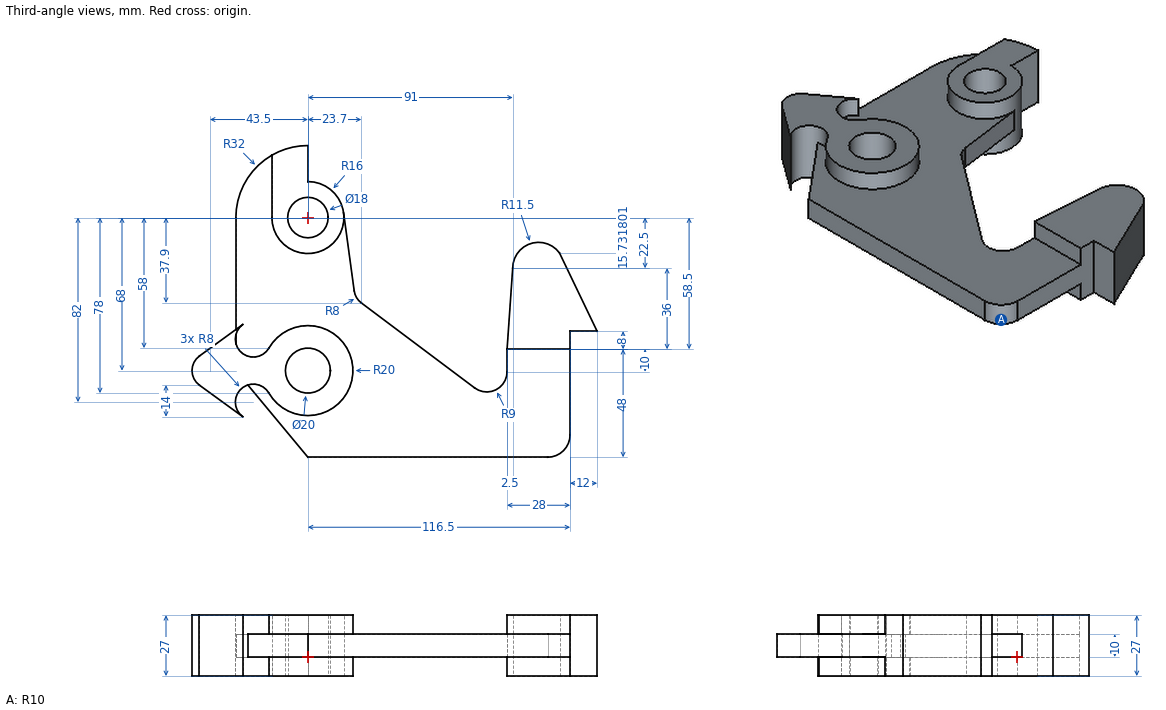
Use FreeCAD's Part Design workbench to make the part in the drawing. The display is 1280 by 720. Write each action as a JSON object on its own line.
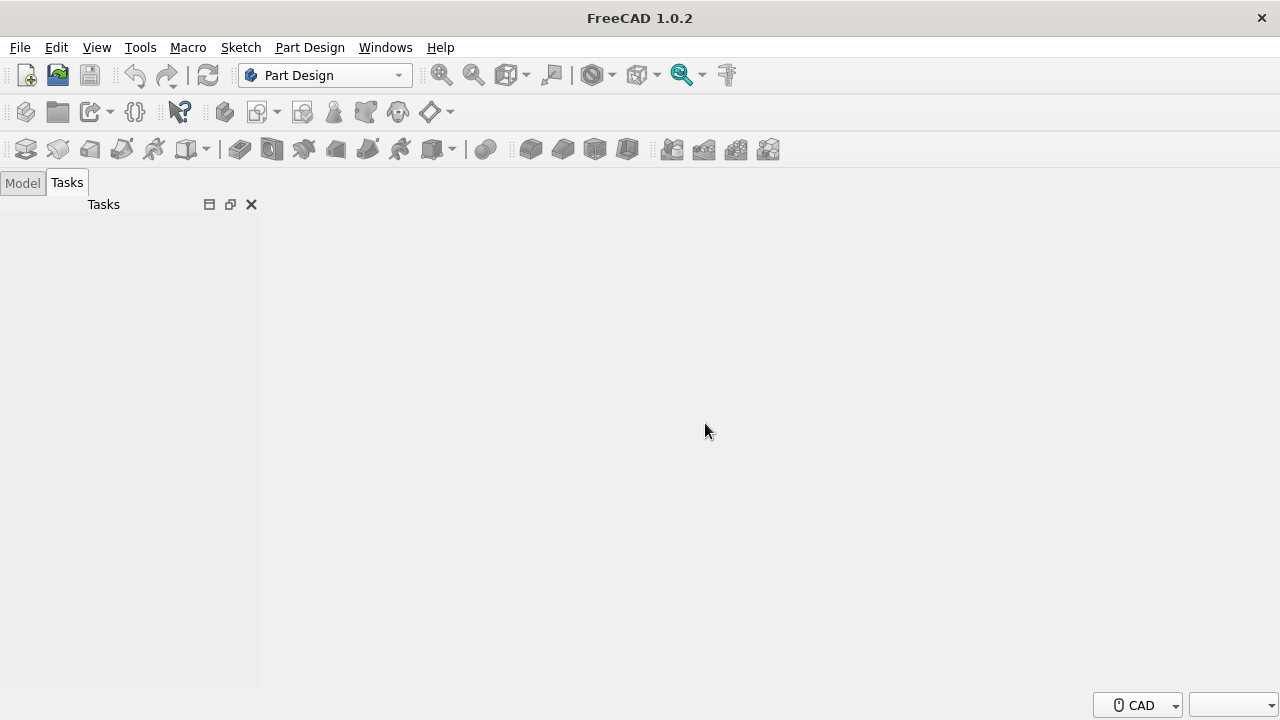
{"action": "left_click", "coordinate": [26, 76]}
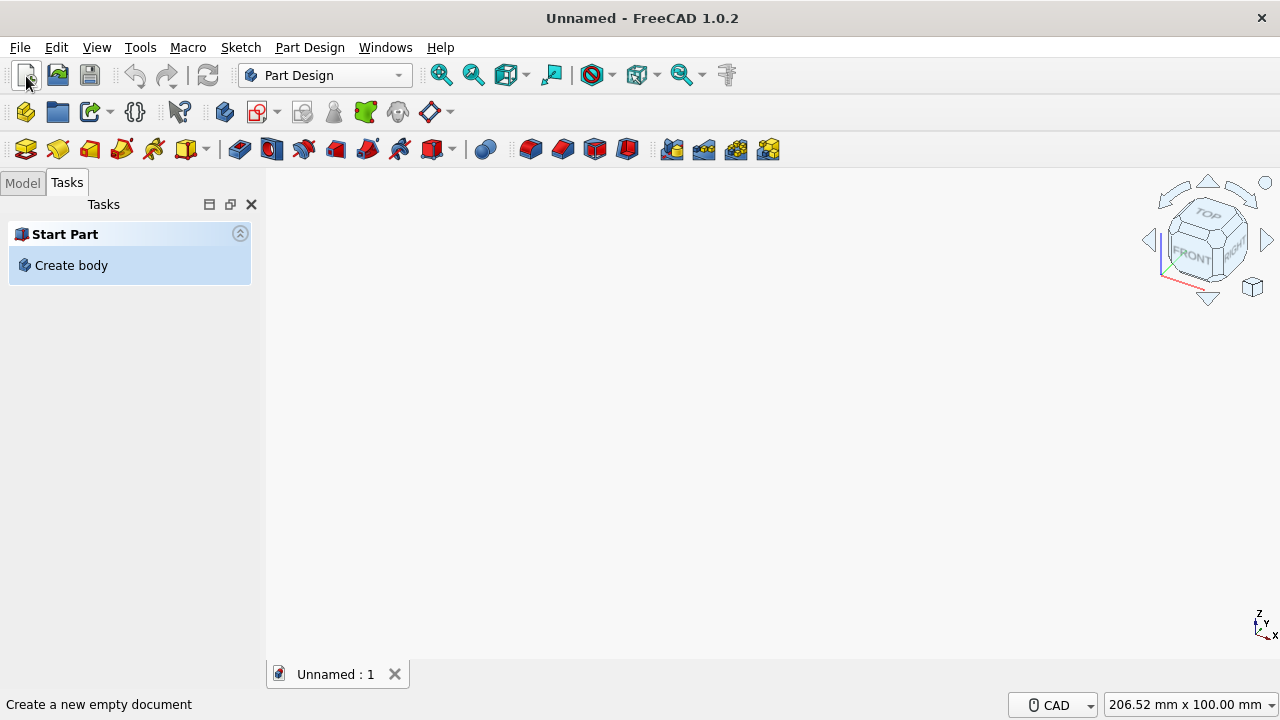
{"action": "left_click", "coordinate": [258, 112]}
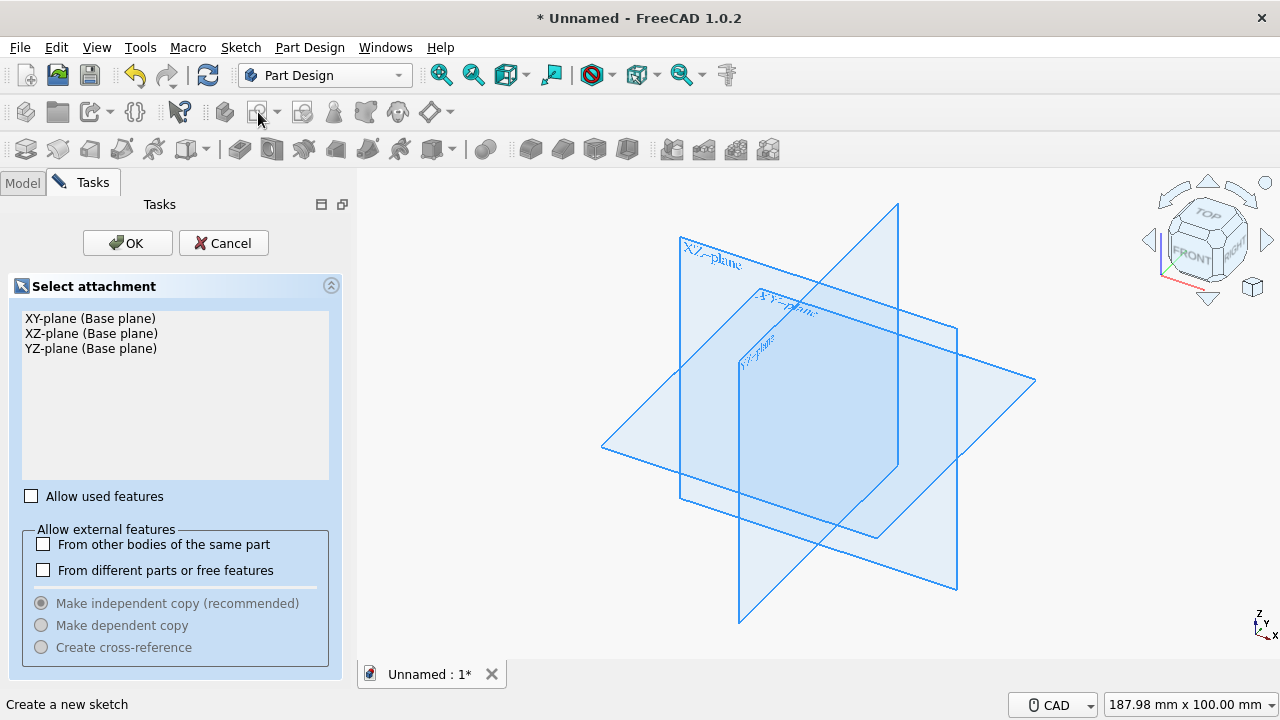
{"action": "left_click", "coordinate": [82, 318]}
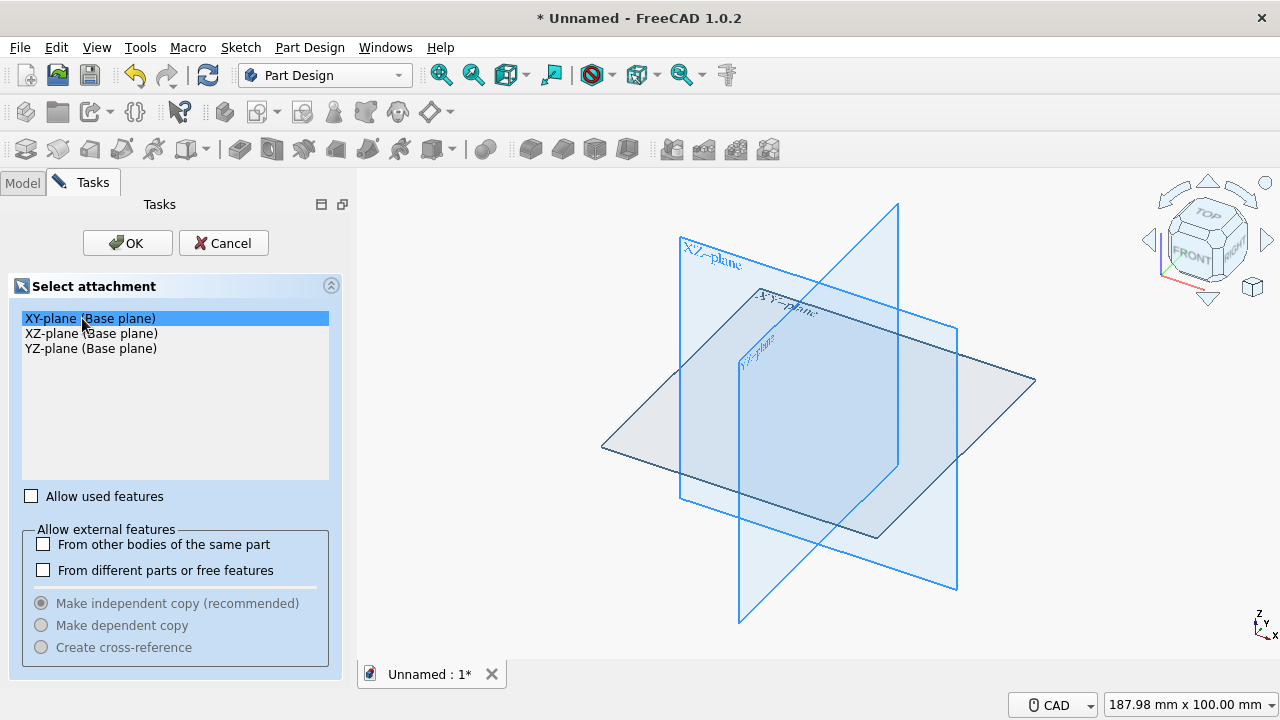
{"action": "left_click", "coordinate": [128, 243]}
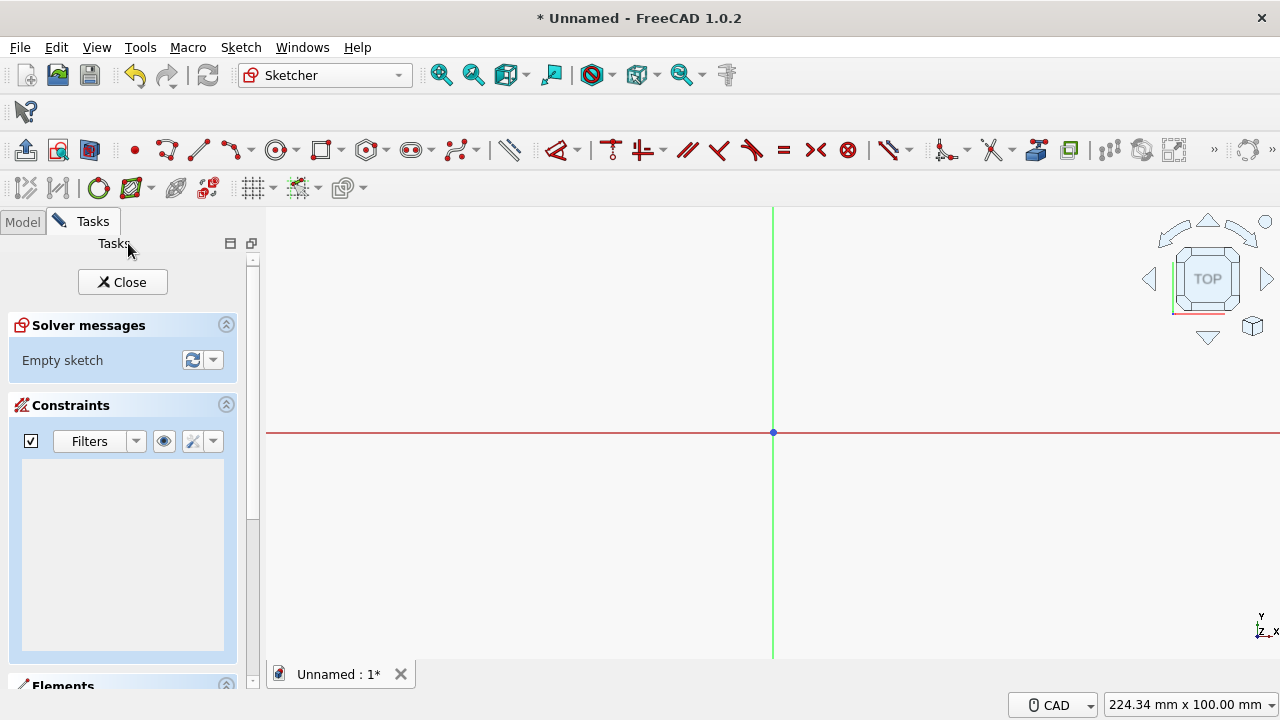
{"action": "scroll", "coordinate": [493, 296], "scroll_direction": "down", "scroll_amount": 4}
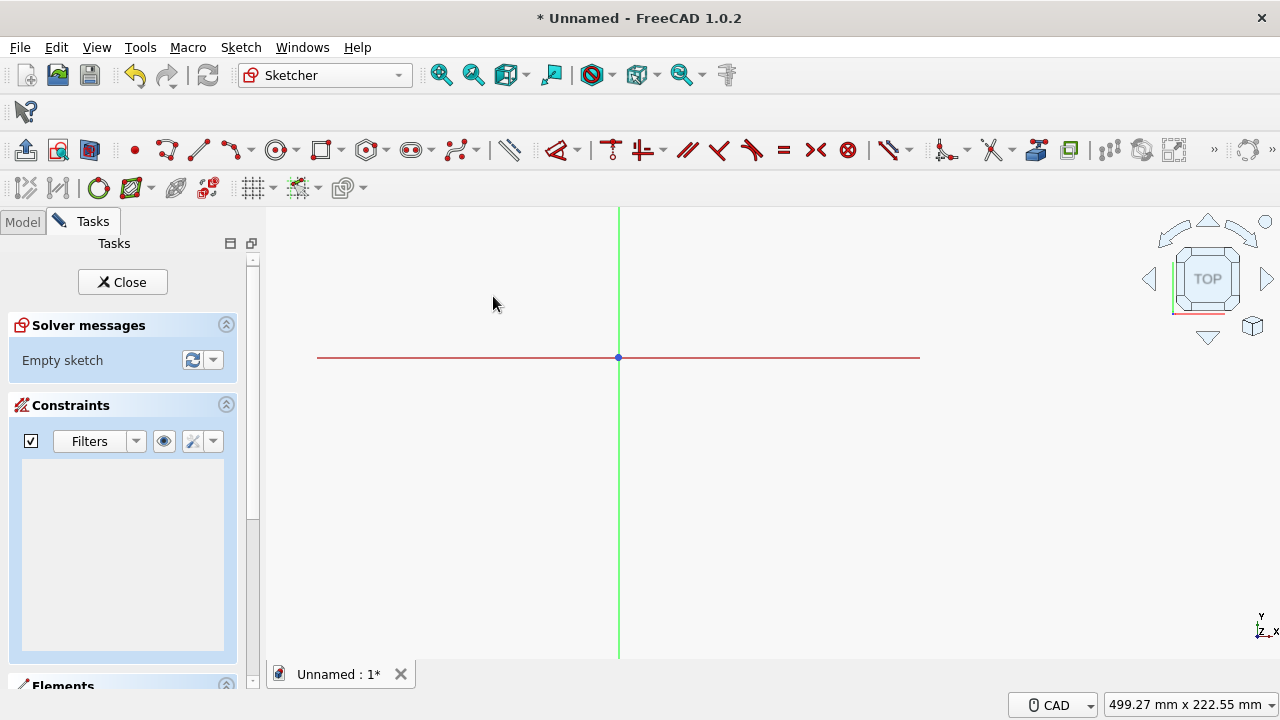
{"action": "left_click", "coordinate": [168, 150]}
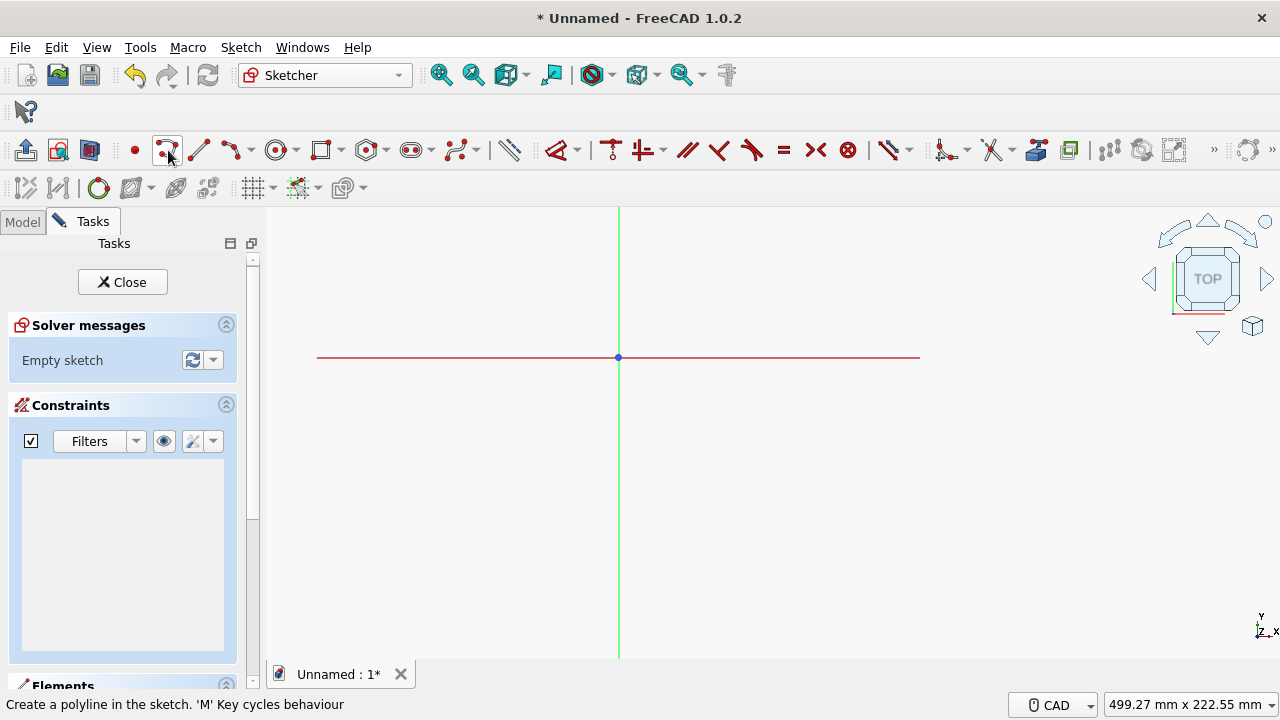
{"action": "left_click", "coordinate": [554, 358]}
{"action": "left_click", "coordinate": [554, 496]}
{"action": "left_click", "coordinate": [619, 574]}
{"action": "left_click", "coordinate": [856, 574]}
{"action": "left_click", "coordinate": [856, 476]}
{"action": "left_click", "coordinate": [799, 476]}
{"action": "left_click", "coordinate": [799, 497]}
{"action": "right_click", "coordinate": [799, 497]}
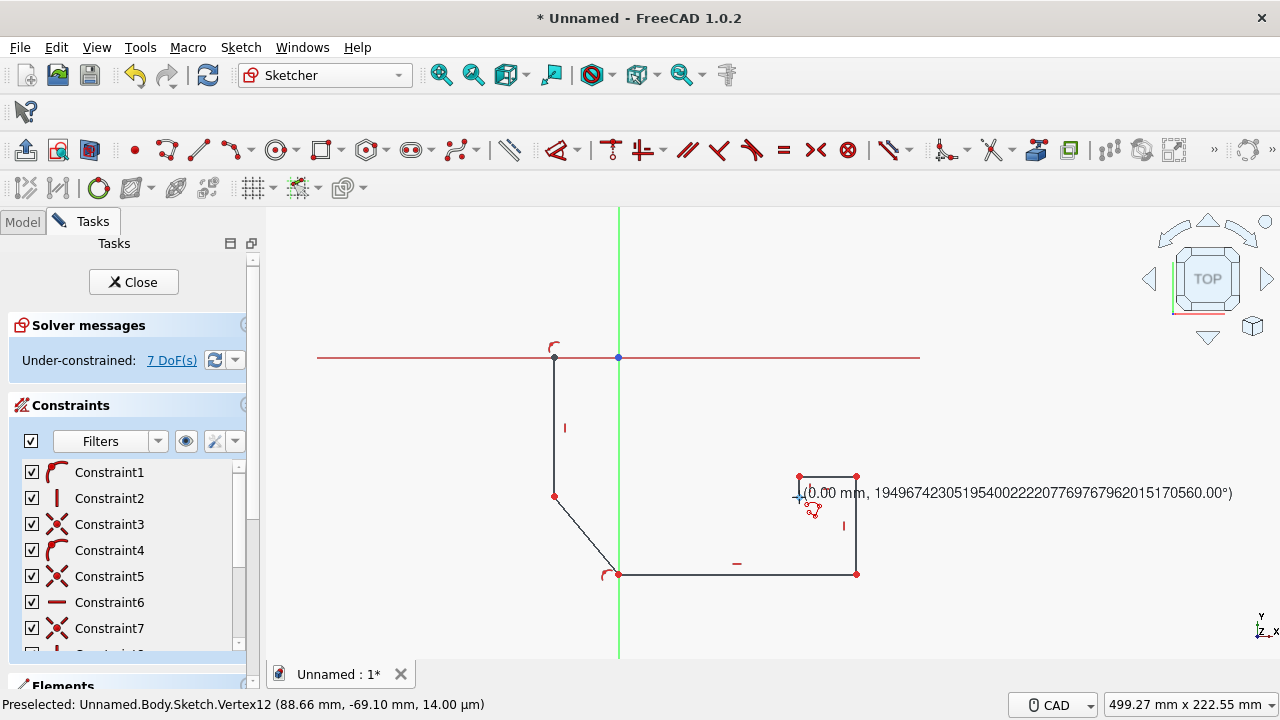
{"action": "left_click", "coordinate": [200, 150]}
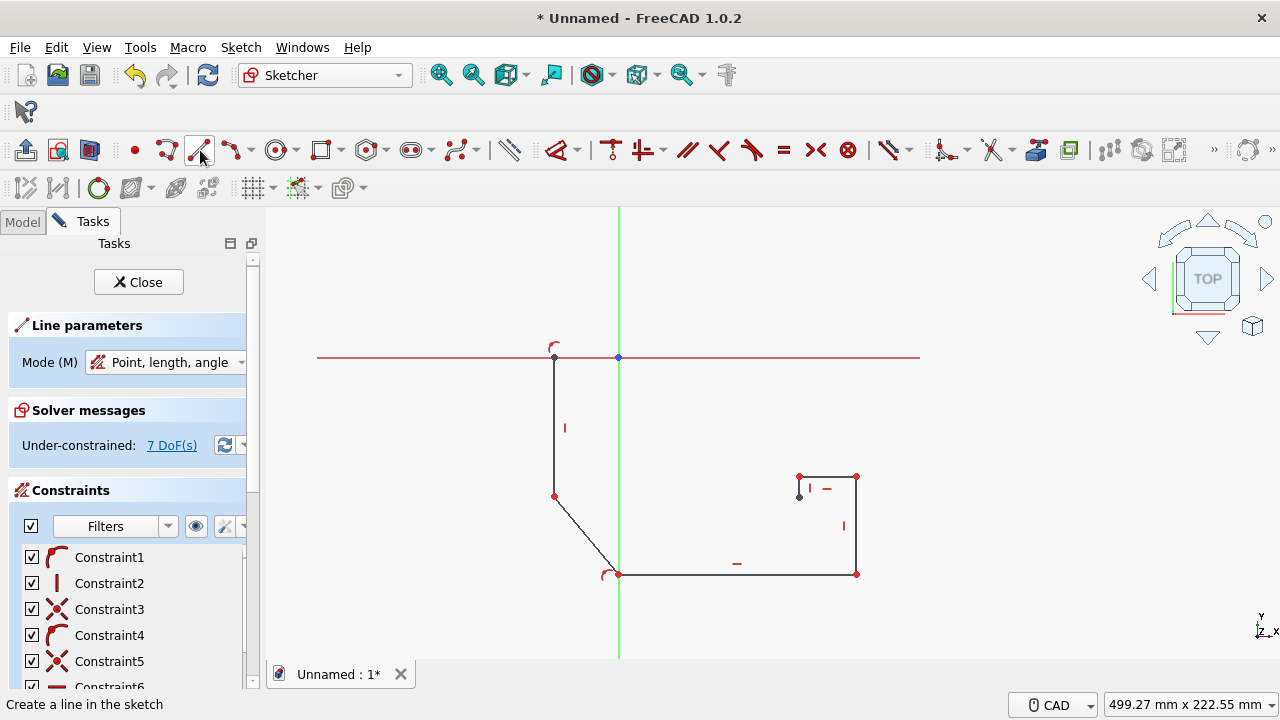
{"action": "left_click", "coordinate": [769, 511]}
{"action": "left_click", "coordinate": [667, 435]}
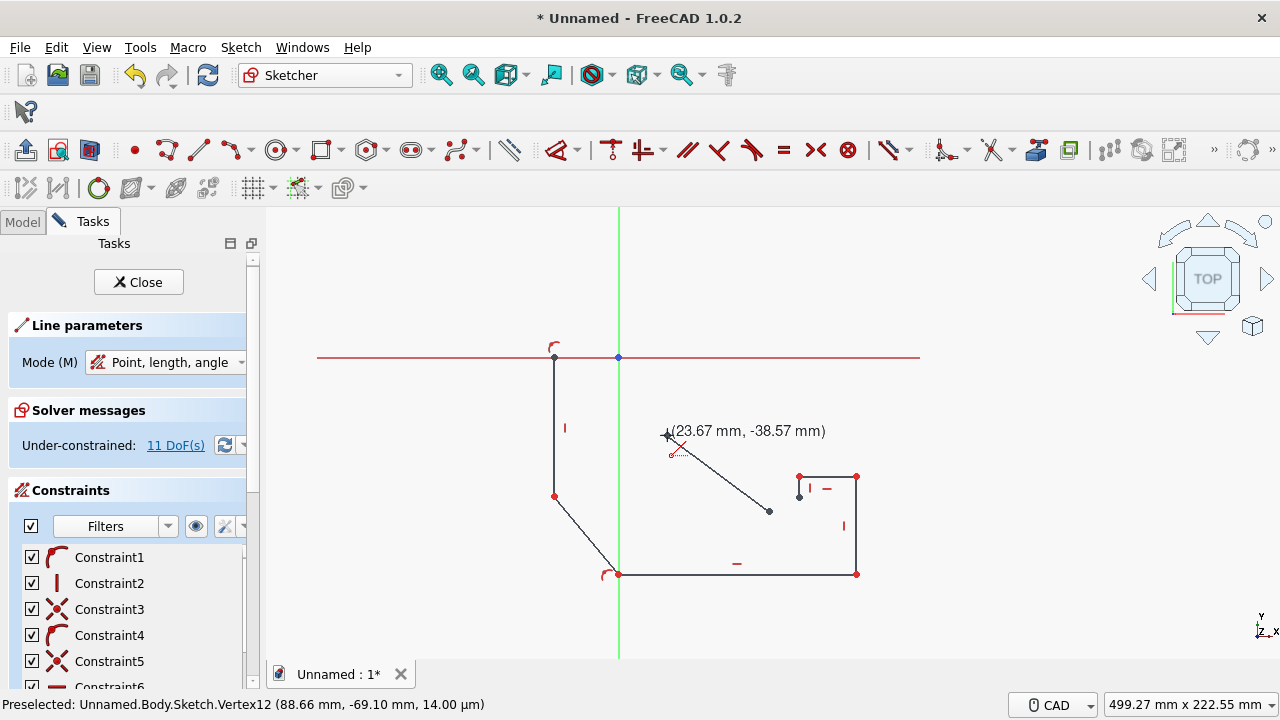
{"action": "scroll", "coordinate": [661, 424], "scroll_direction": "up", "scroll_amount": 2}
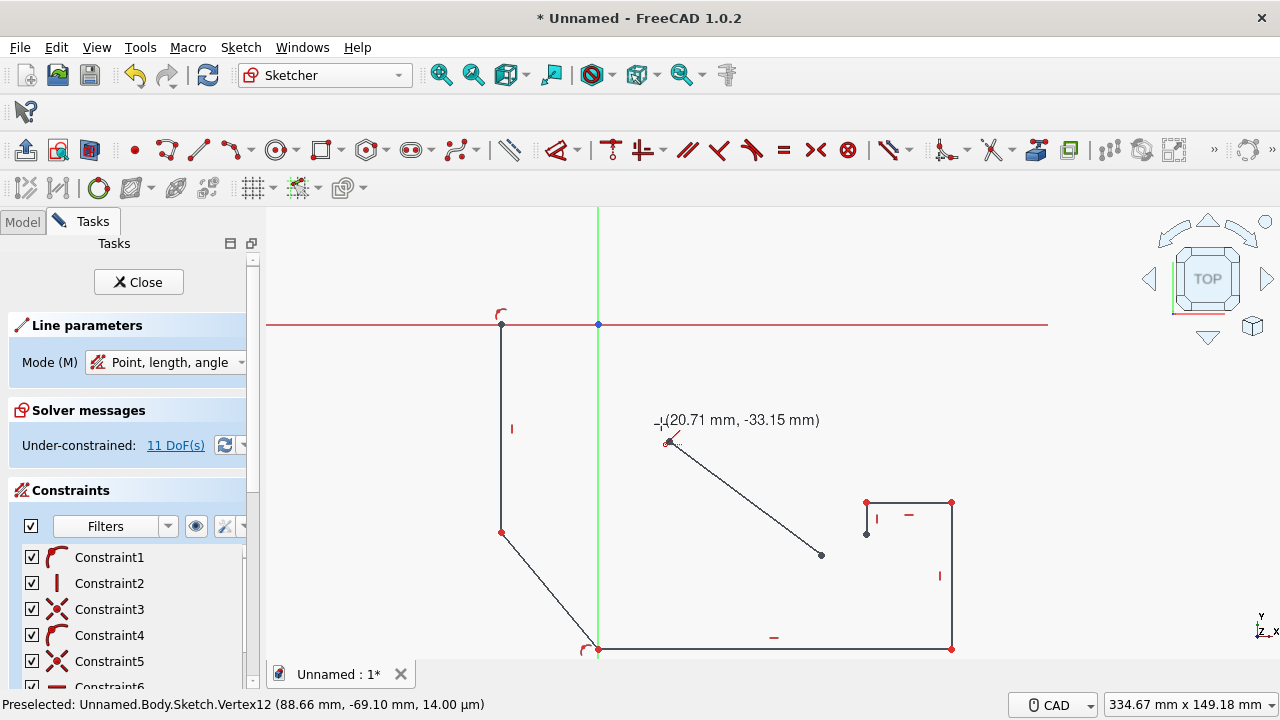
{"action": "left_click", "coordinate": [660, 424]}